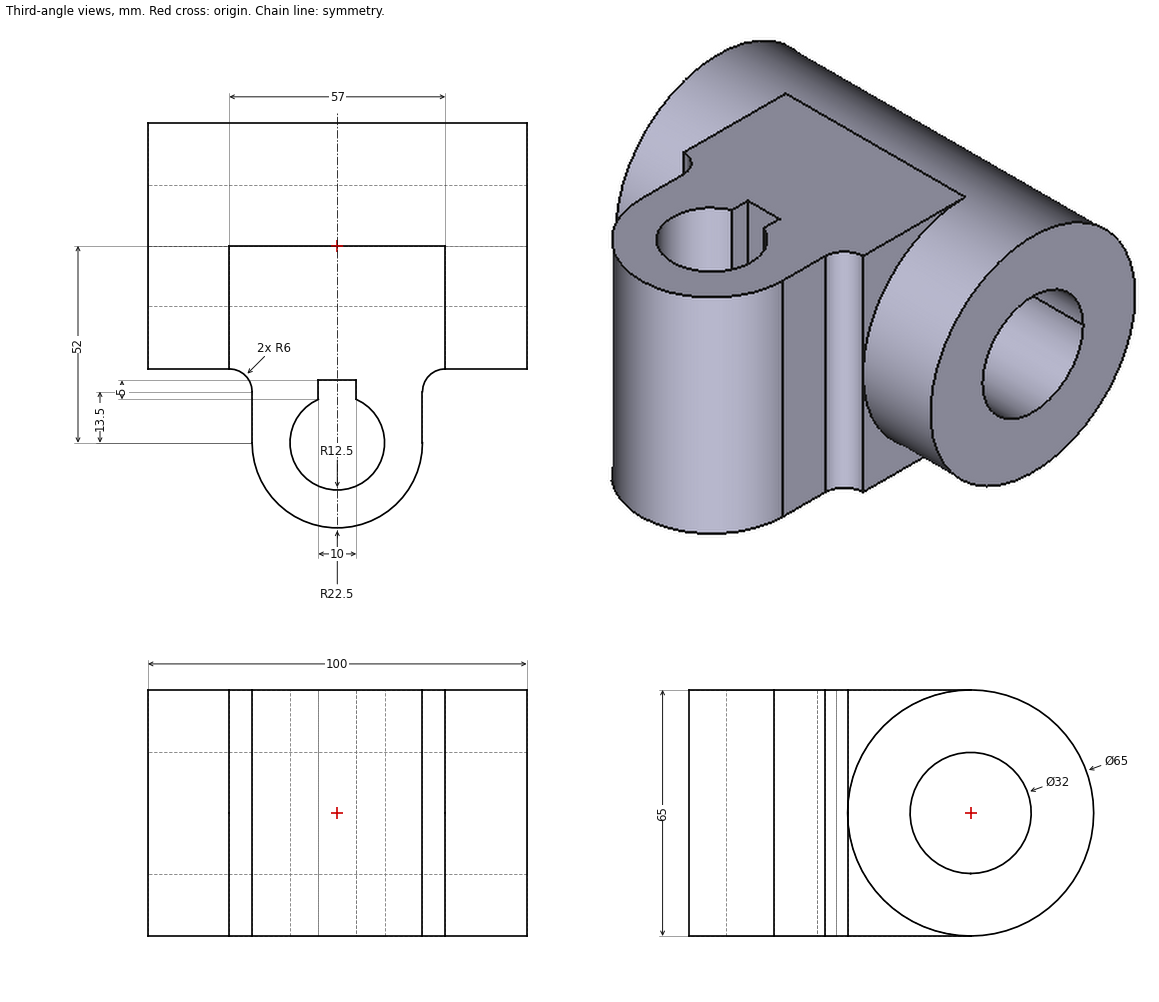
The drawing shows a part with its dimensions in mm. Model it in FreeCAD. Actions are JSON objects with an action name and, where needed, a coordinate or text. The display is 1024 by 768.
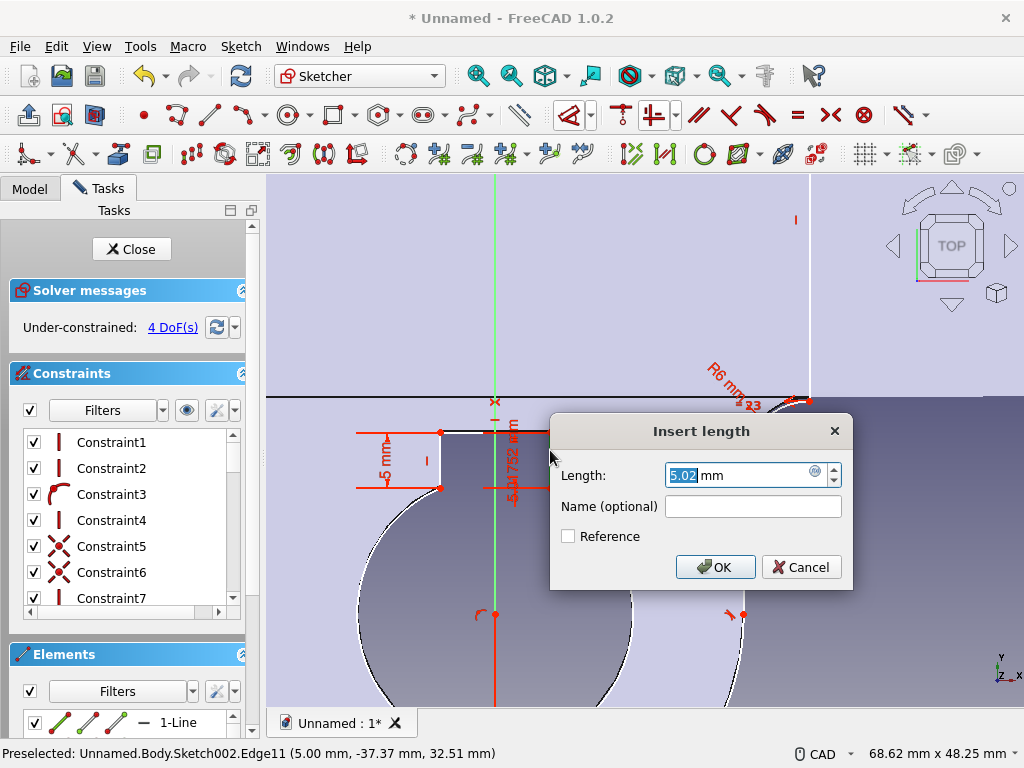
{"action": "type", "text": "5"}
{"action": "key", "text": "Return"}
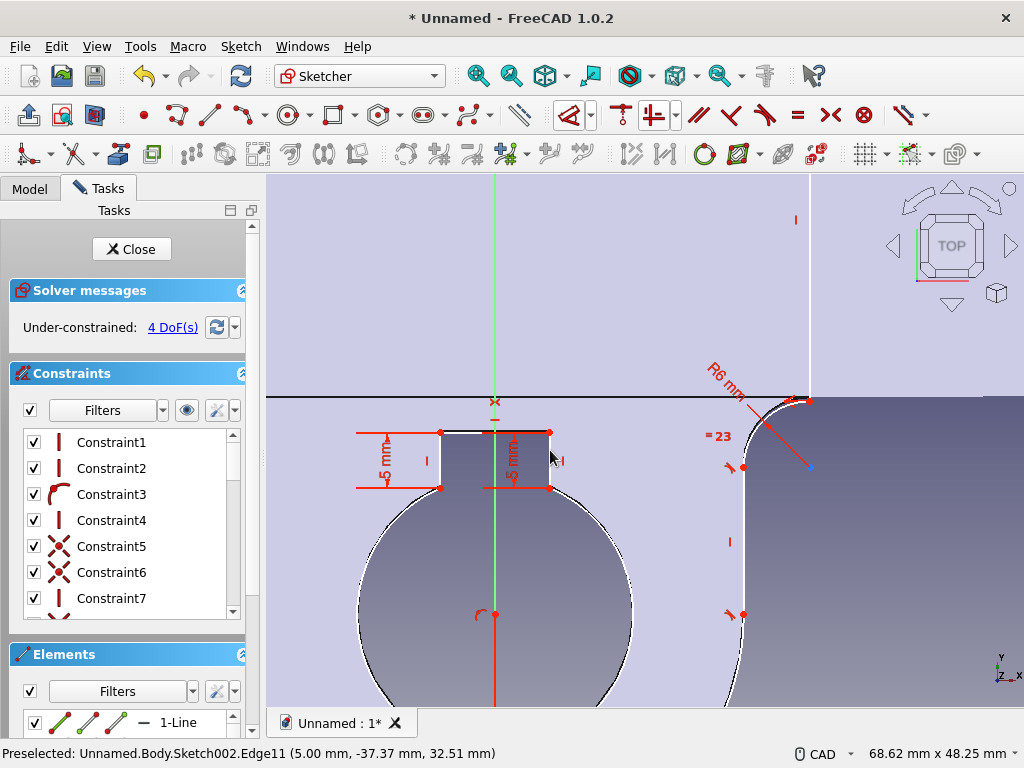
{"action": "scroll", "coordinate": [643, 433], "scroll_direction": "down", "scroll_amount": 4}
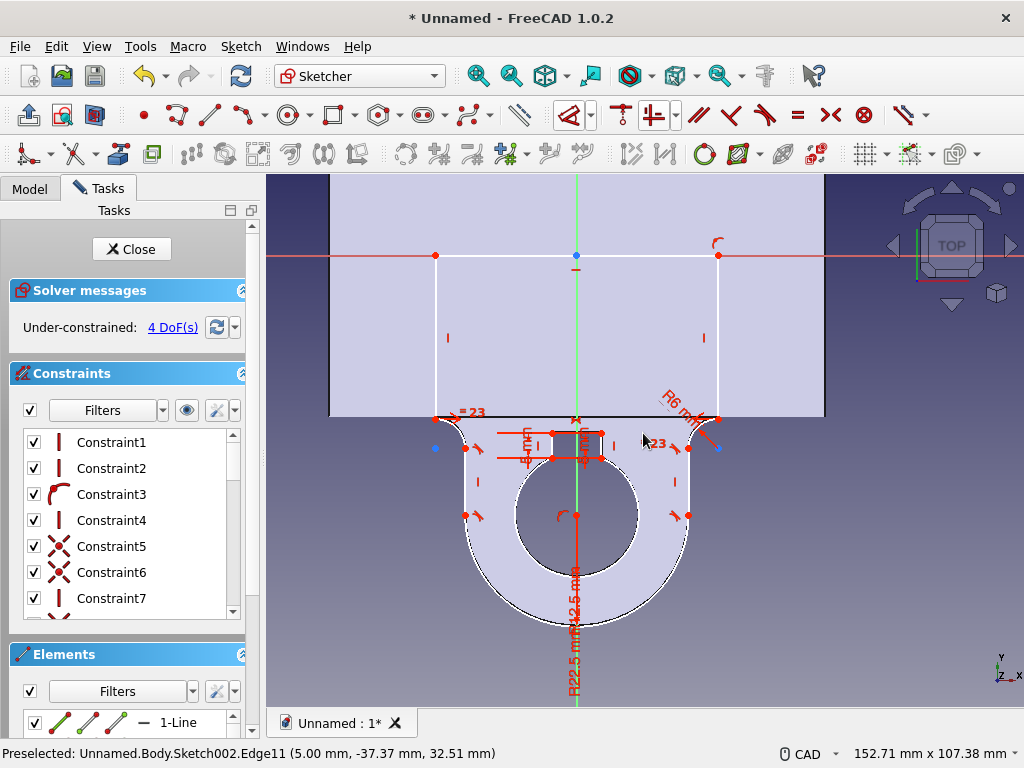
{"action": "left_click", "coordinate": [633, 256]}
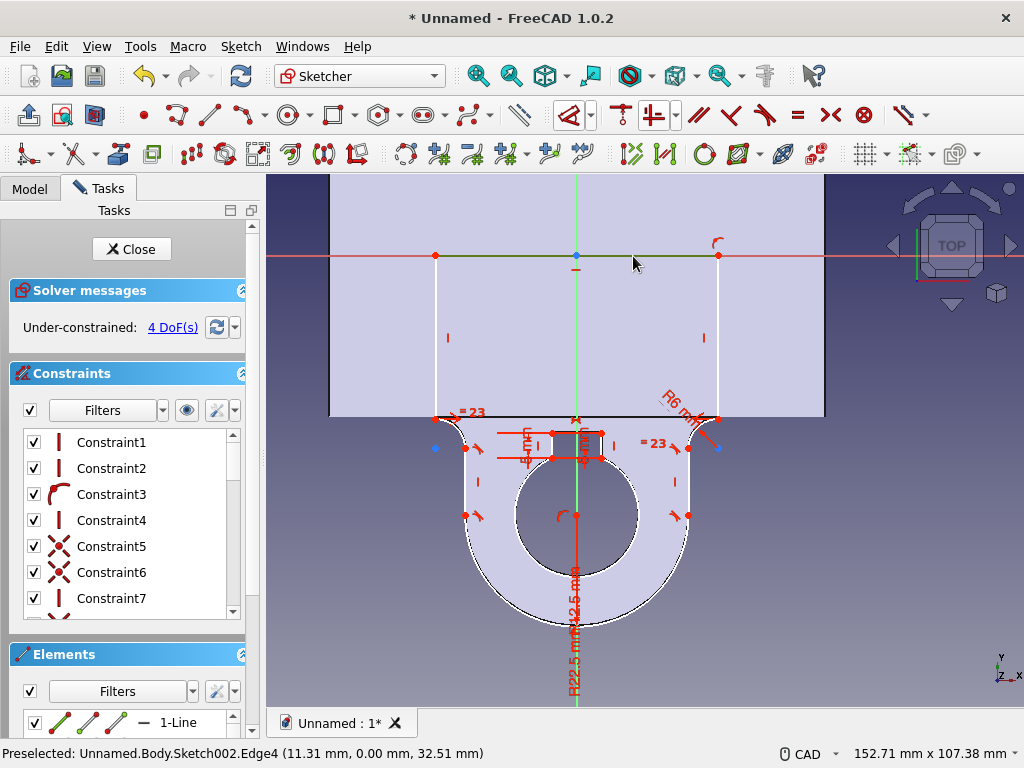
{"action": "key", "text": "l"}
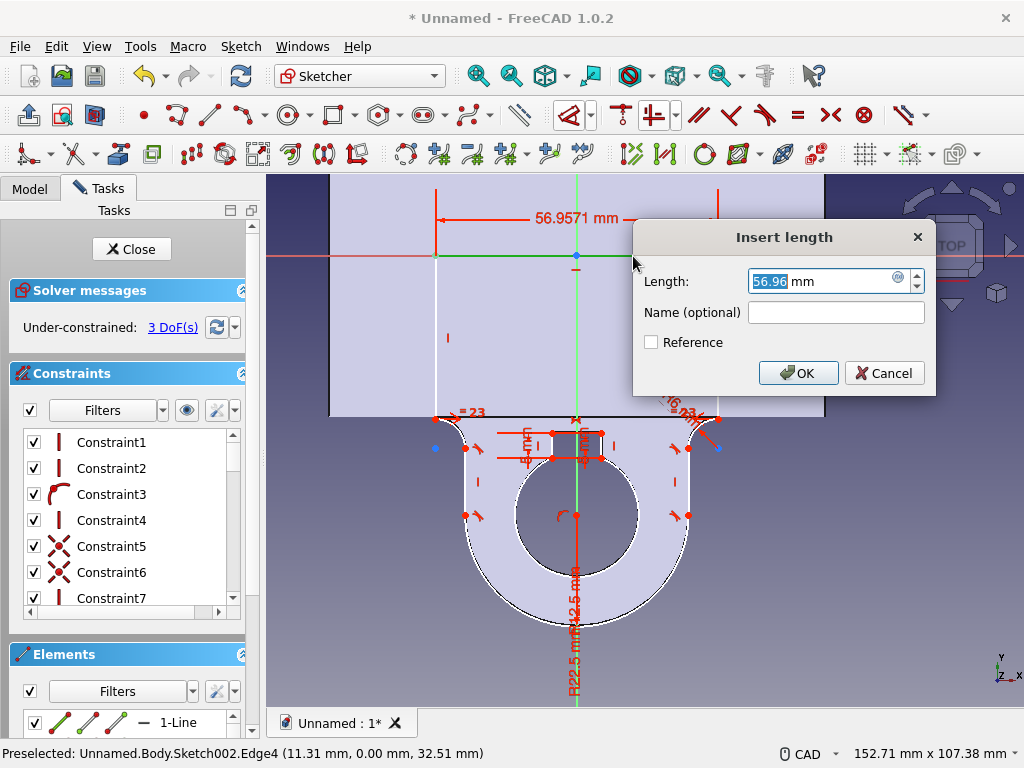
{"action": "type", "text": "57"}
{"action": "key", "text": "Return"}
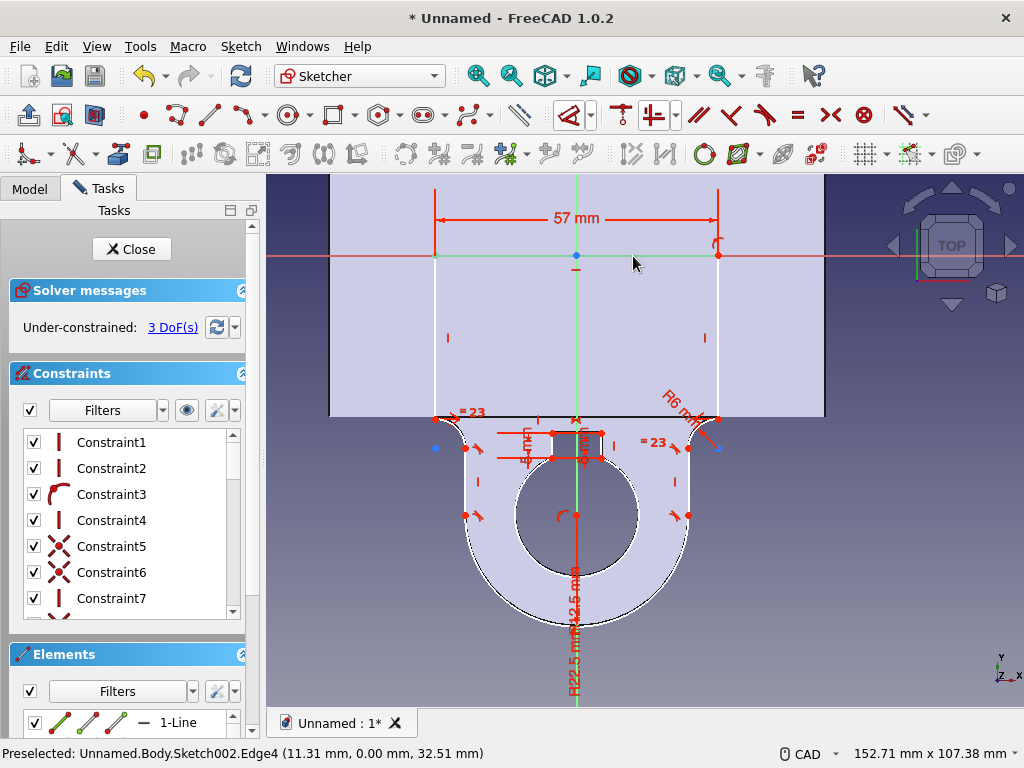
{"action": "scroll", "coordinate": [567, 433], "scroll_direction": "up", "scroll_amount": 2}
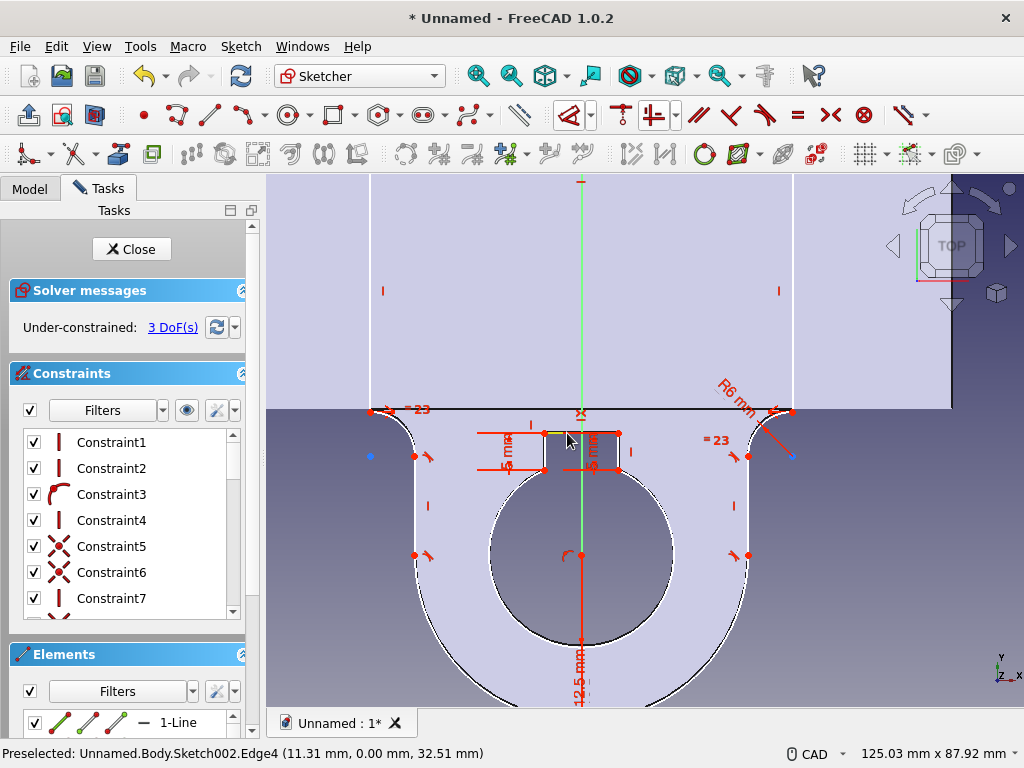
{"action": "left_click", "coordinate": [567, 433]}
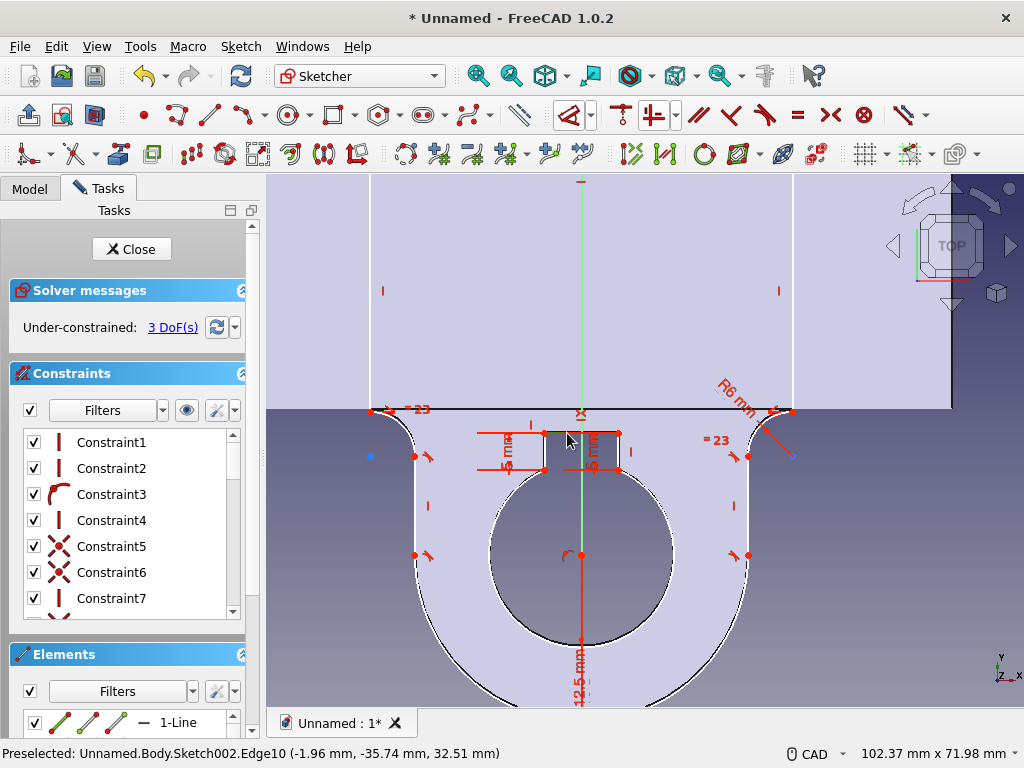
{"action": "key", "text": "l"}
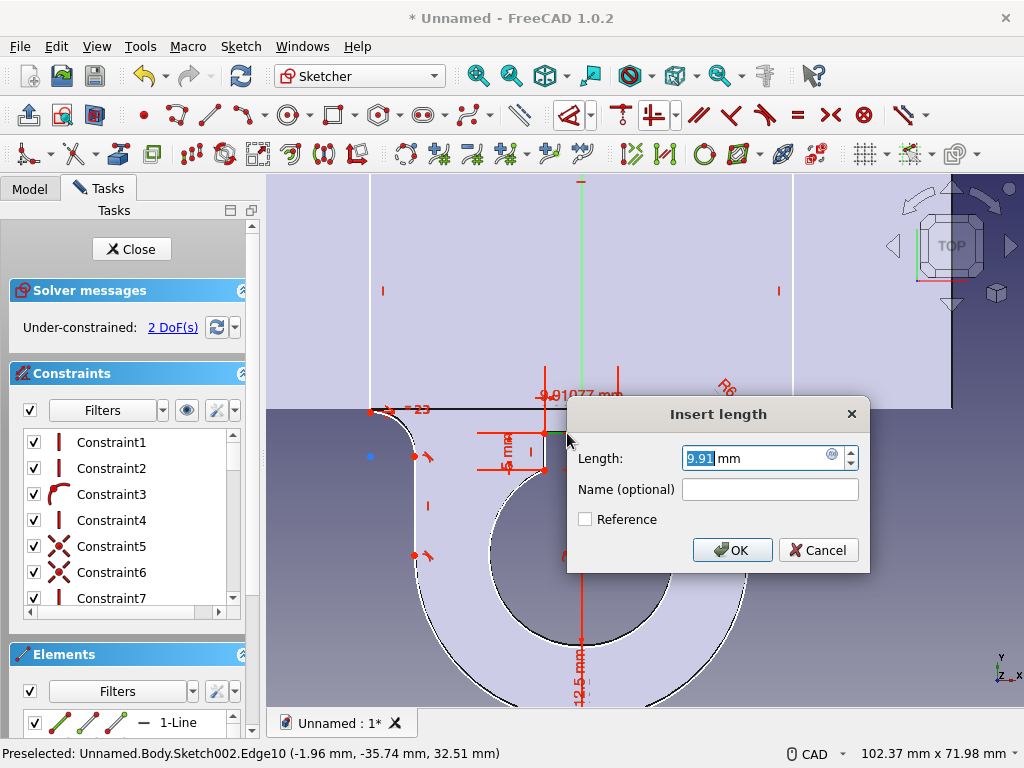
{"action": "type", "text": "10"}
{"action": "key", "text": "Return"}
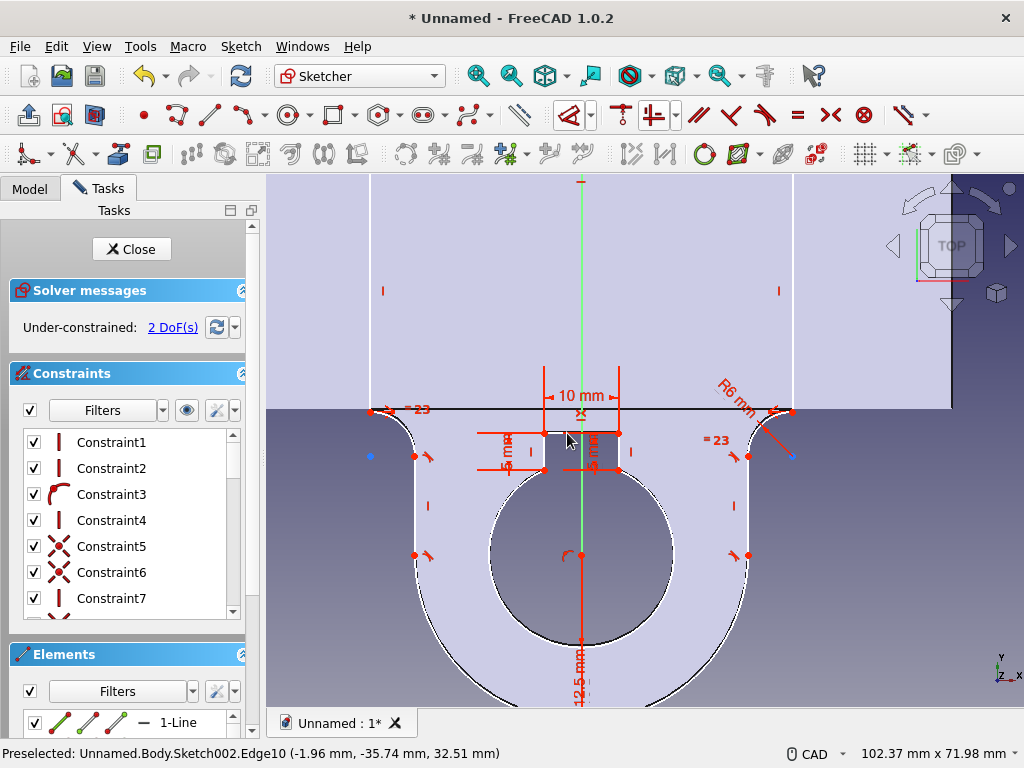
{"action": "left_click", "coordinate": [415, 555]}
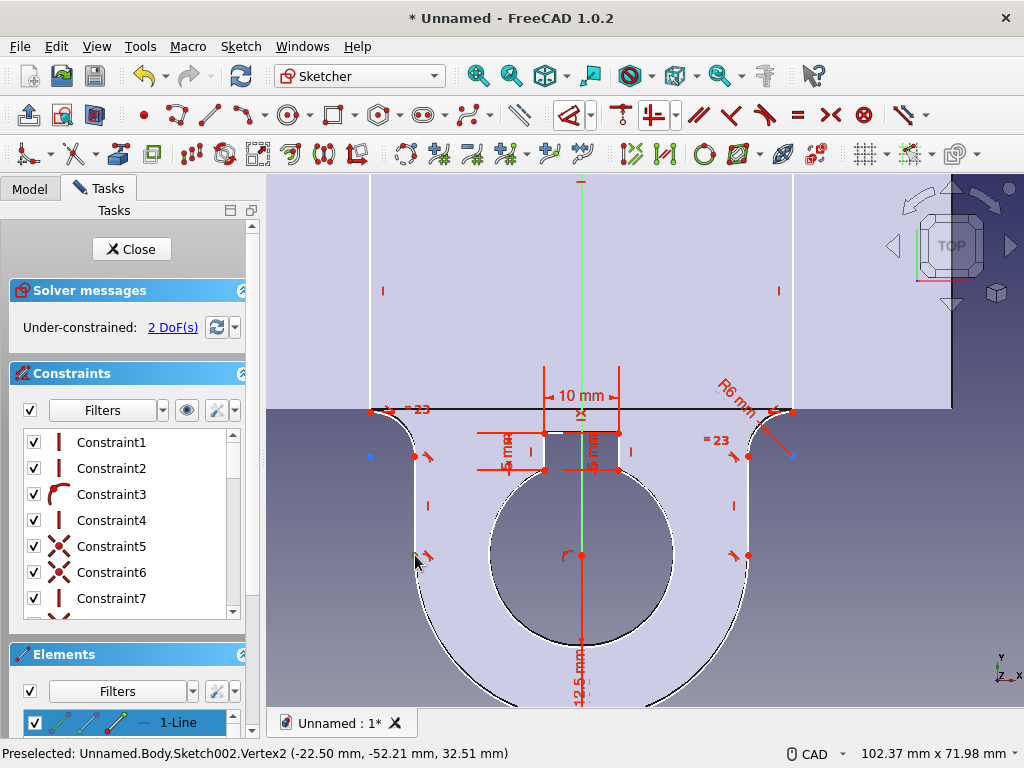
{"action": "key", "text": "i"}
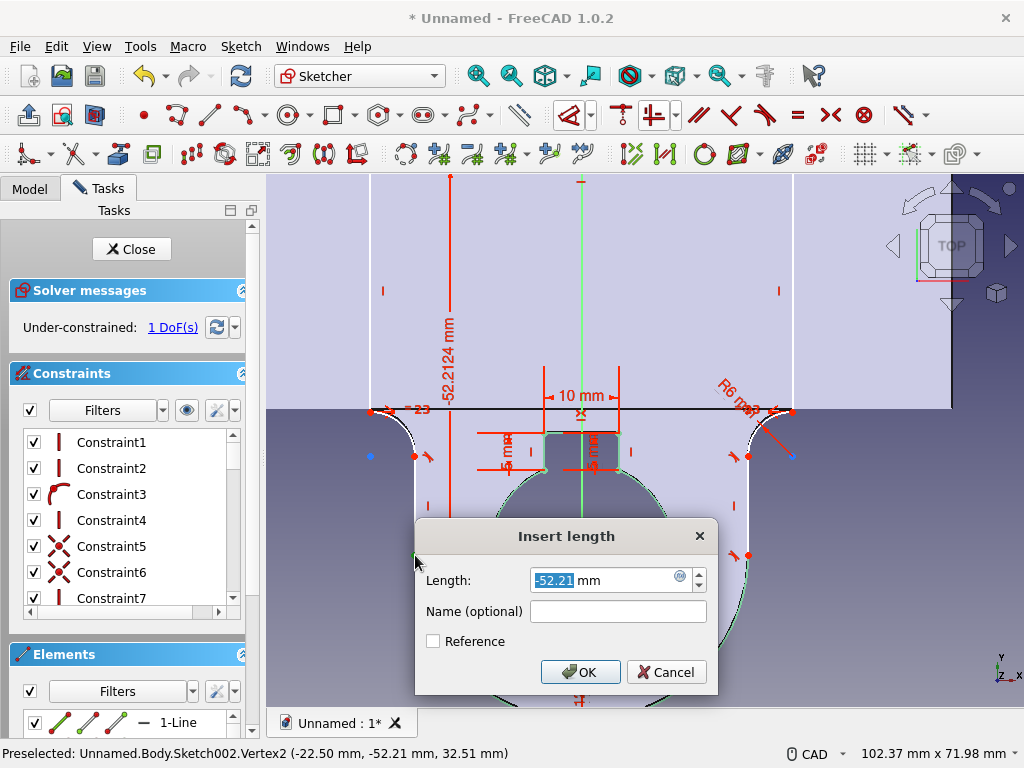
{"action": "type", "text": "-52"}
{"action": "key", "text": "Return"}